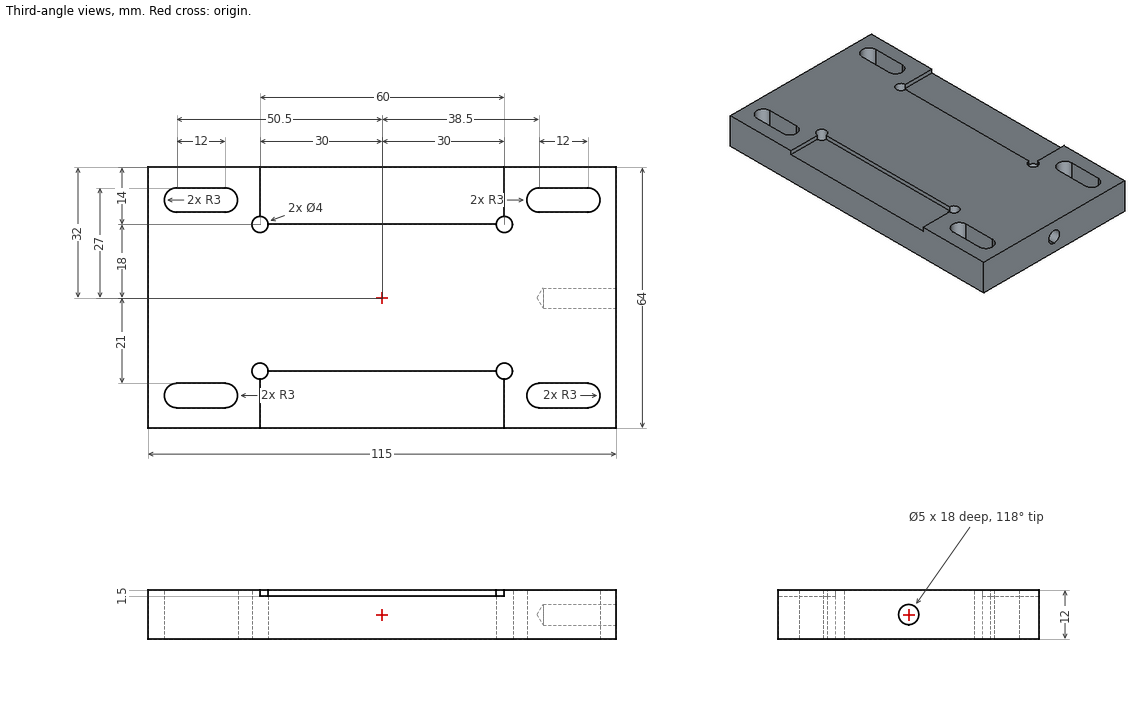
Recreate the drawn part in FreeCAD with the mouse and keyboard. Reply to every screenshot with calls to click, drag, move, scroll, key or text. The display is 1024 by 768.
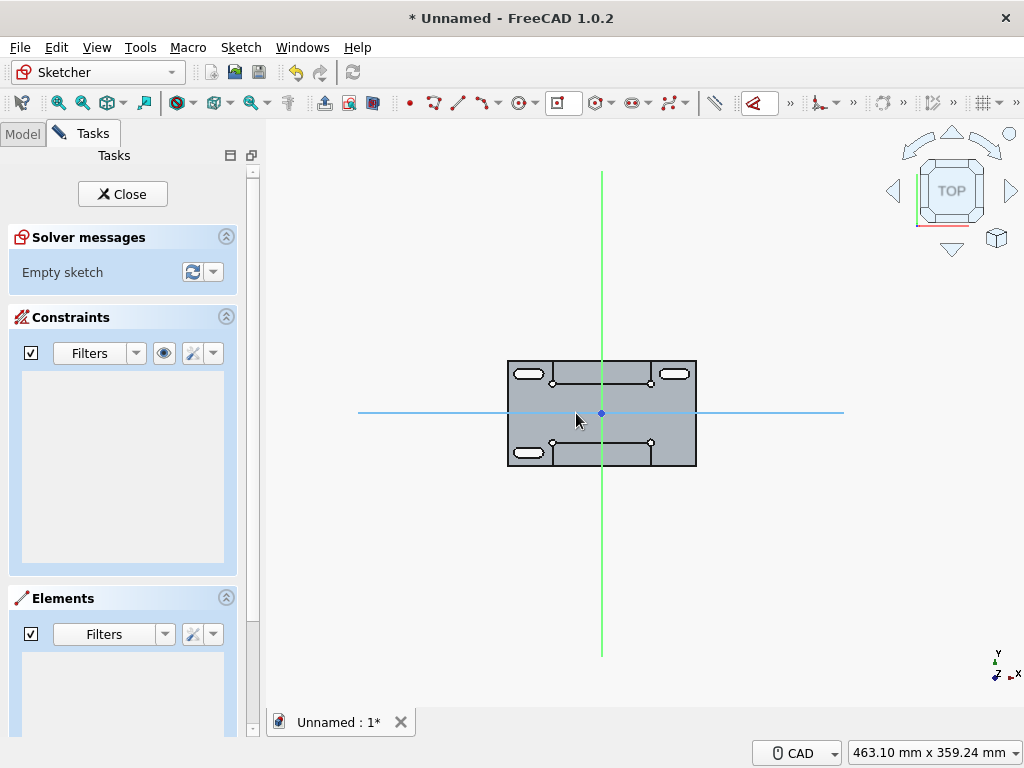
scroll(682, 456, up, 13)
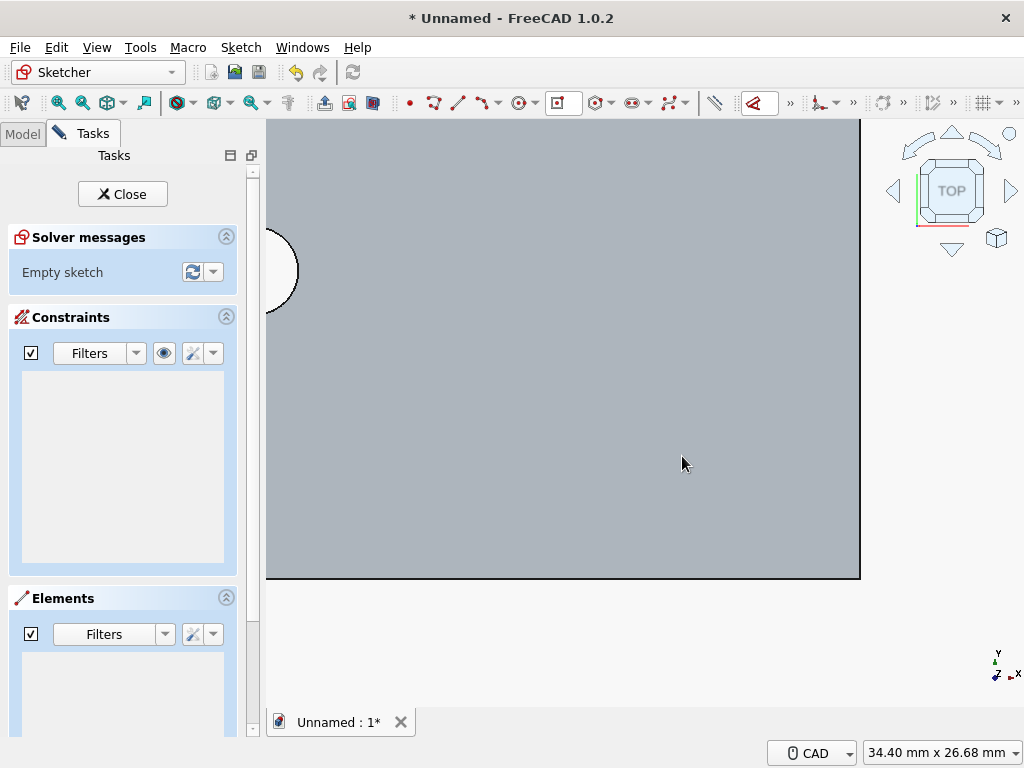
click(632, 104)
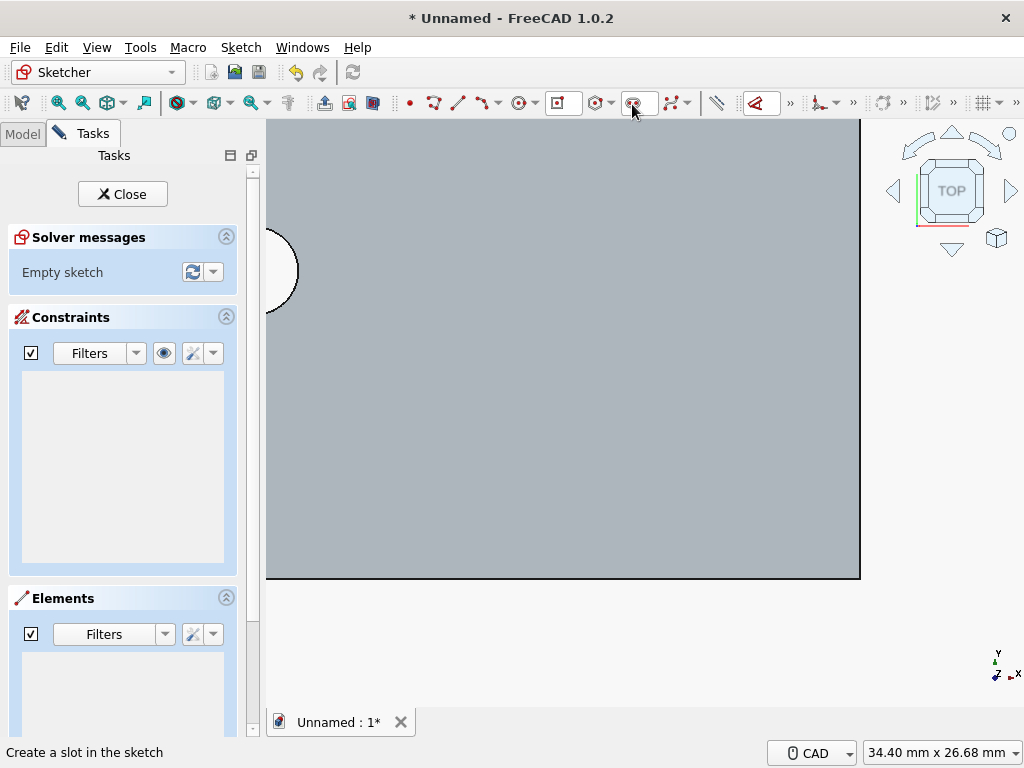
click(442, 403)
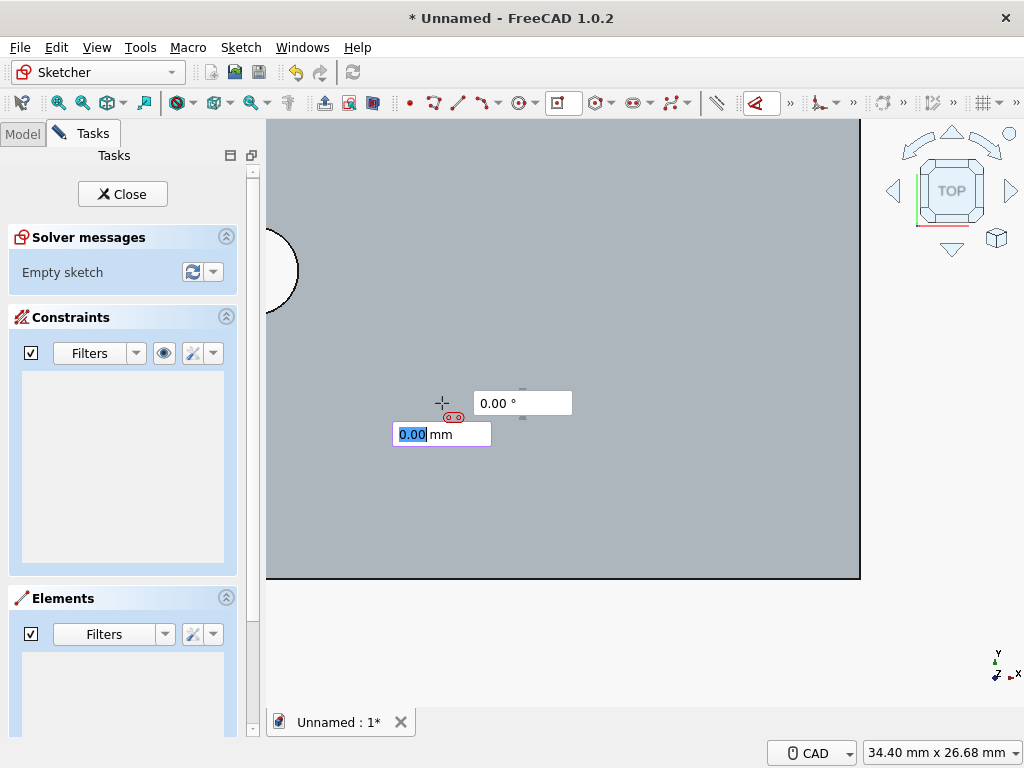
click(706, 403)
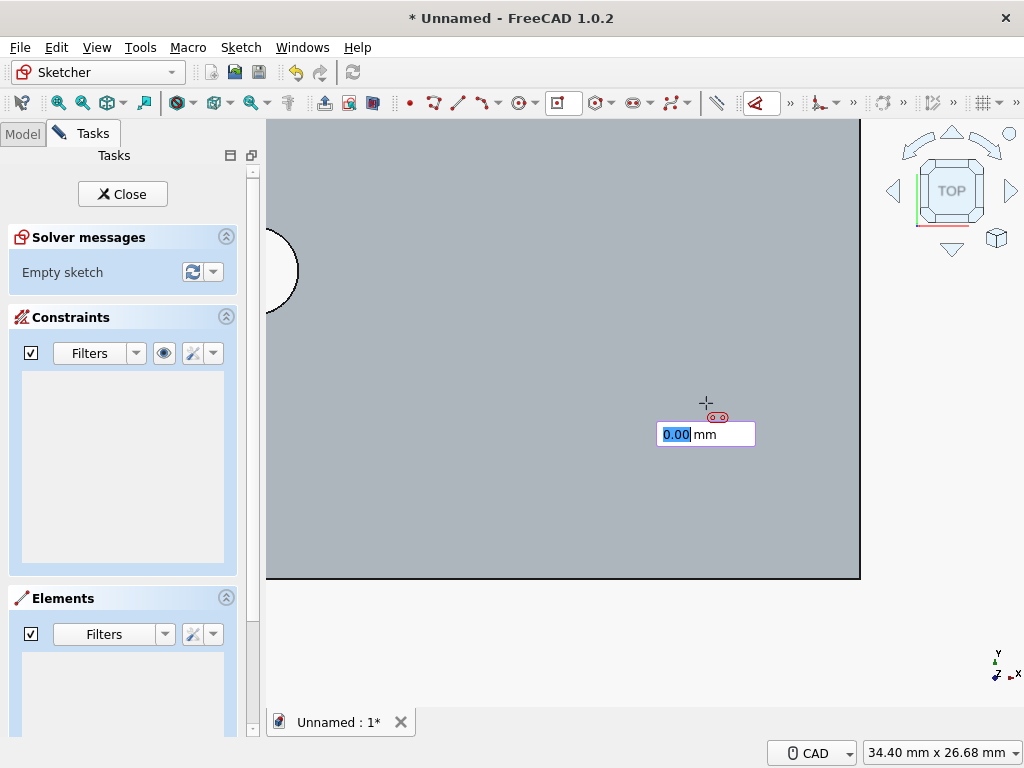
click(574, 469)
key(Escape)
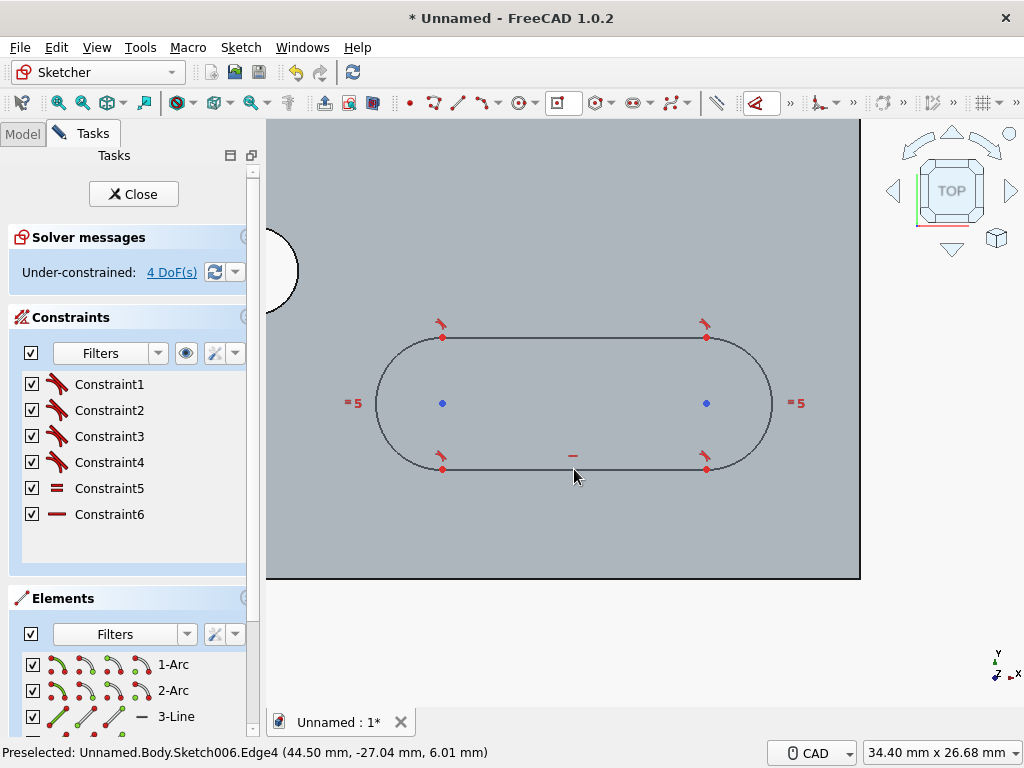
click(389, 365)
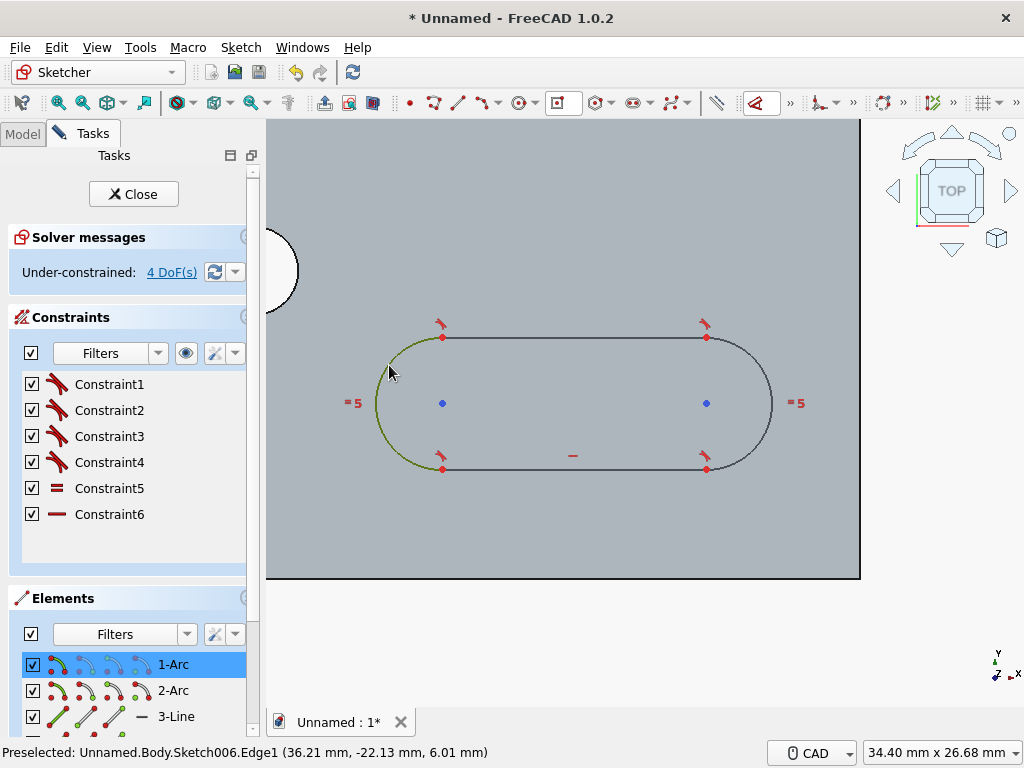
click(774, 104)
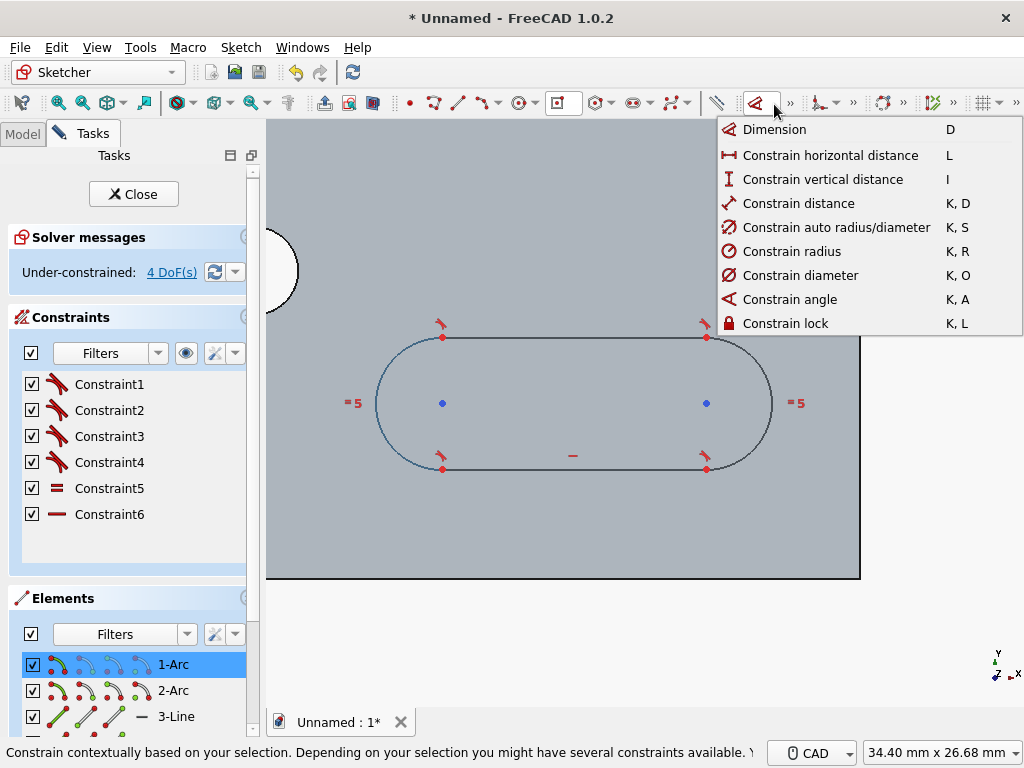
click(870, 251)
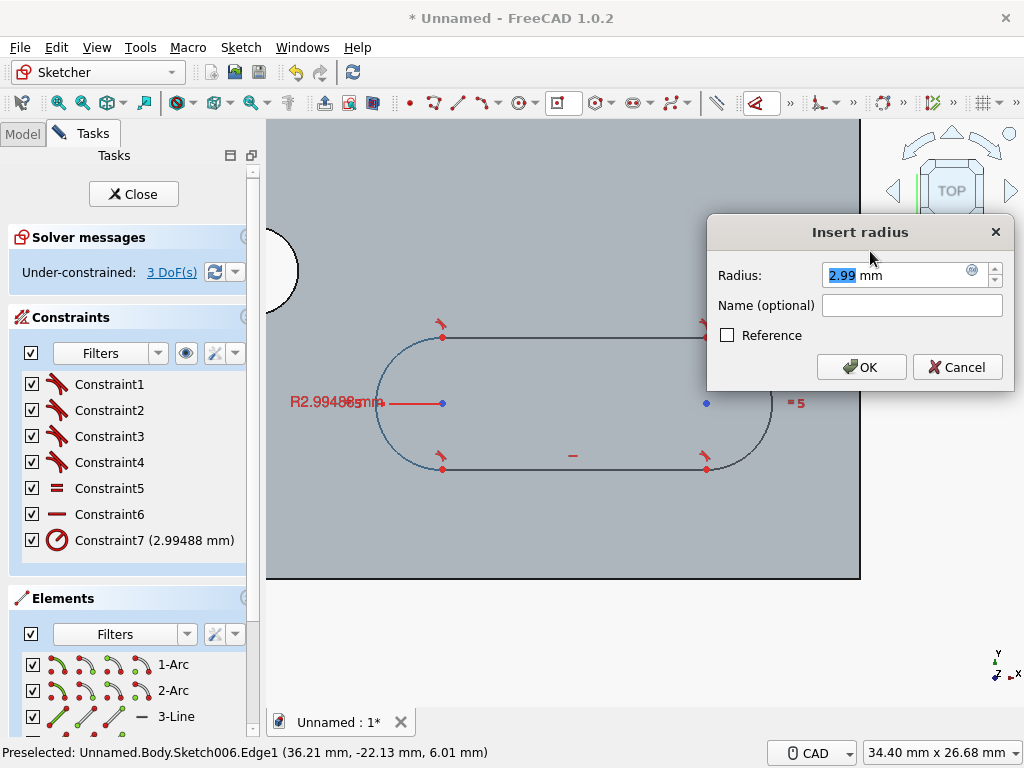
text(3)
key(Return)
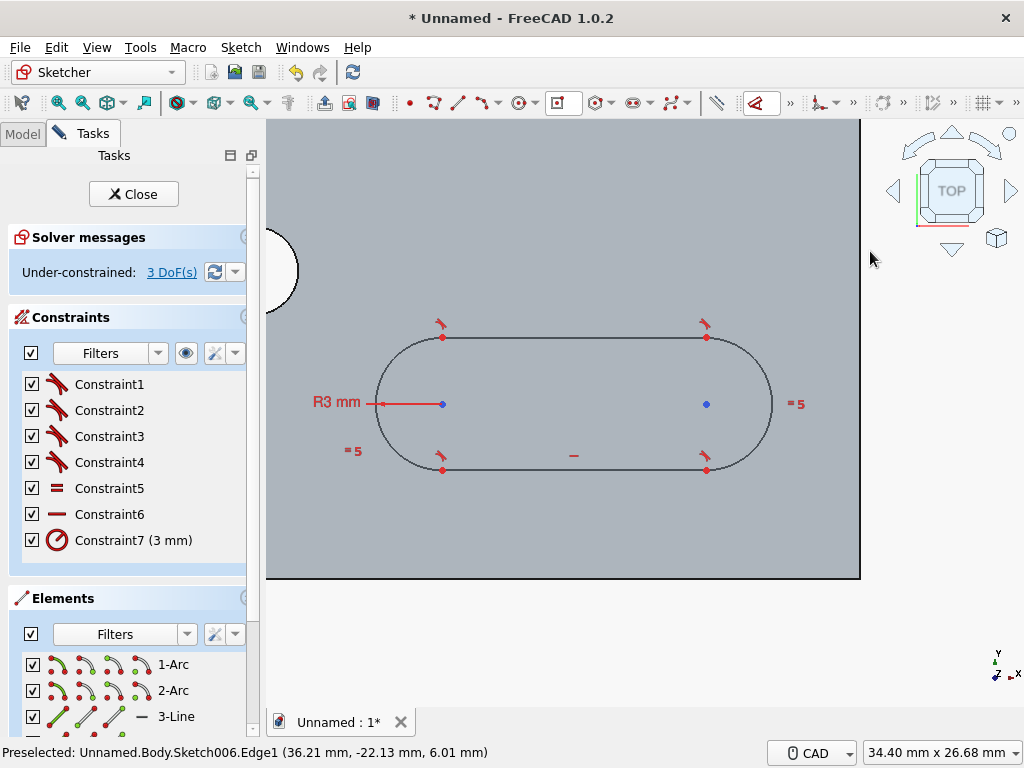
click(521, 338)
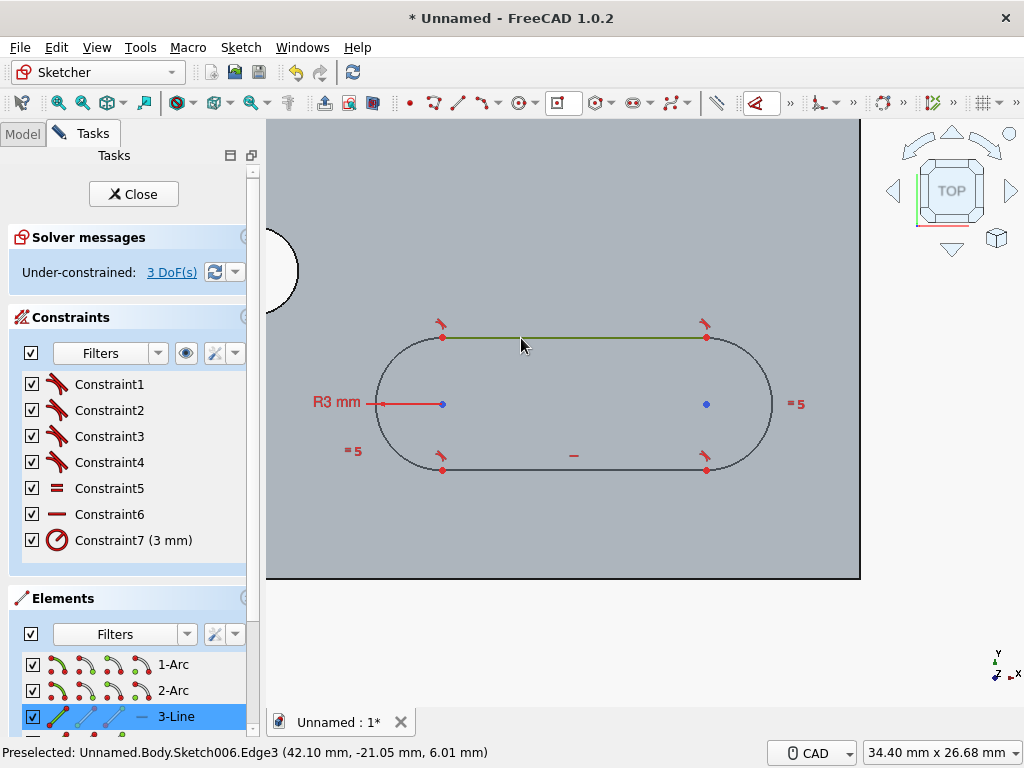
key(l)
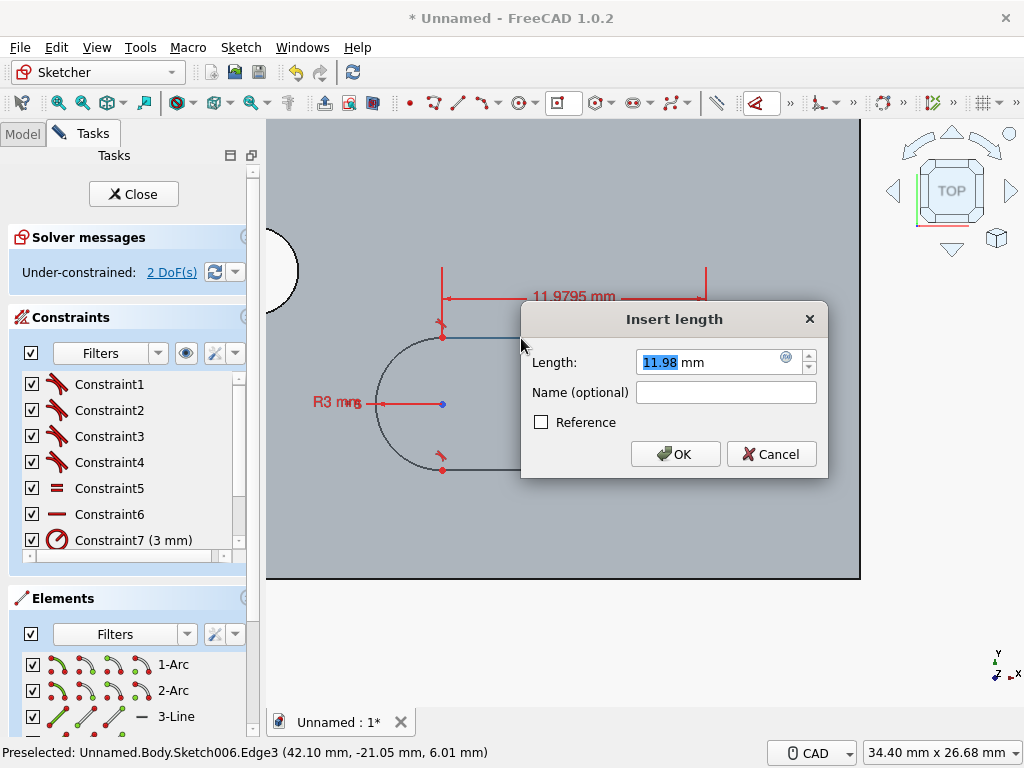
text(12)
key(Return)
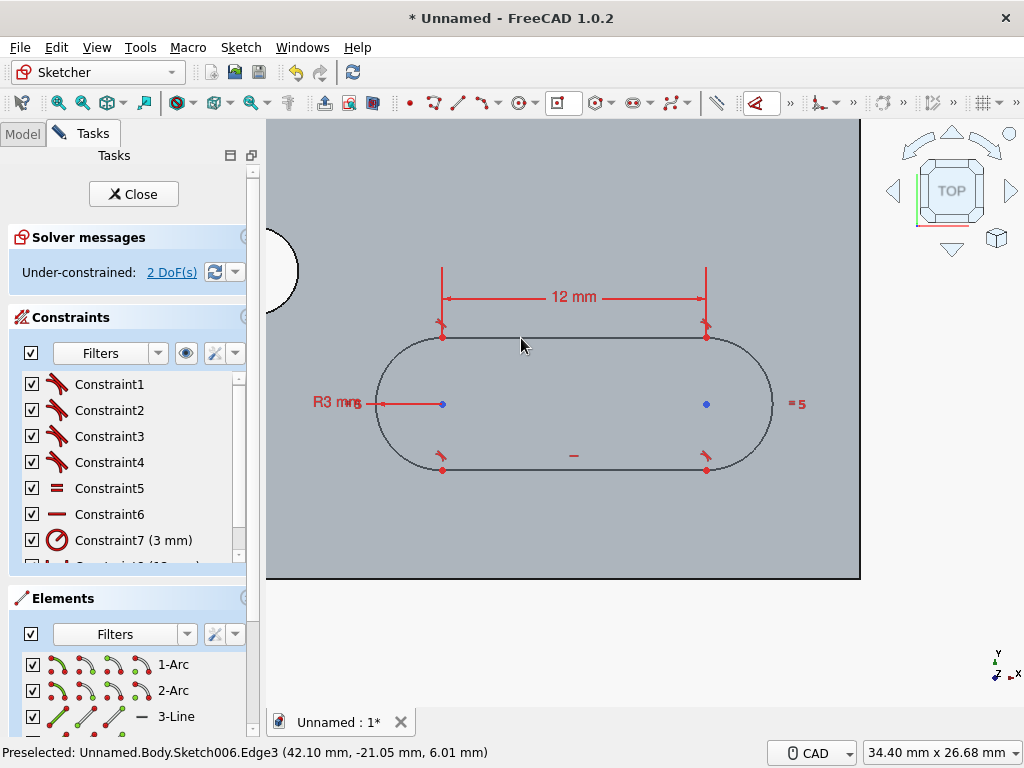
click(442, 338)